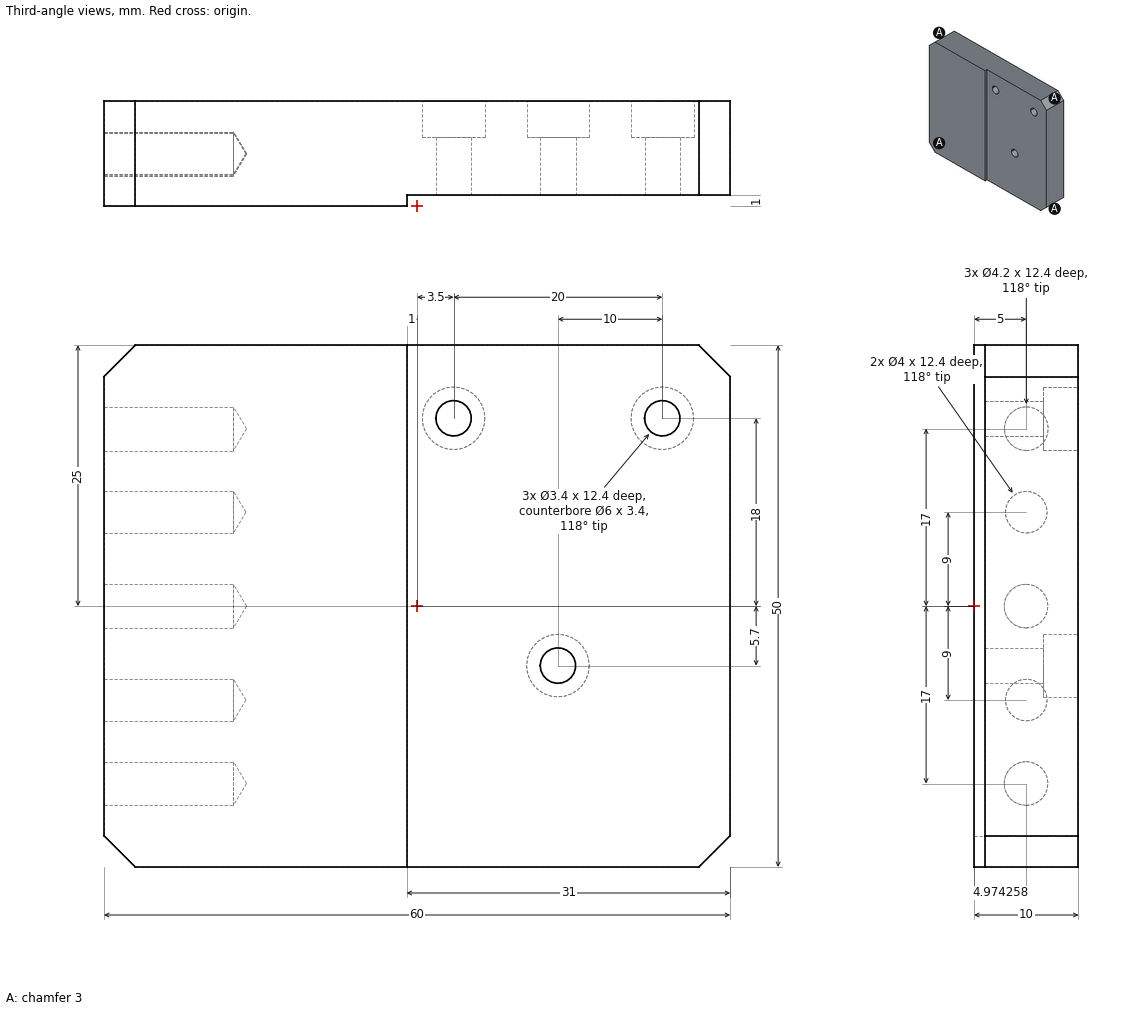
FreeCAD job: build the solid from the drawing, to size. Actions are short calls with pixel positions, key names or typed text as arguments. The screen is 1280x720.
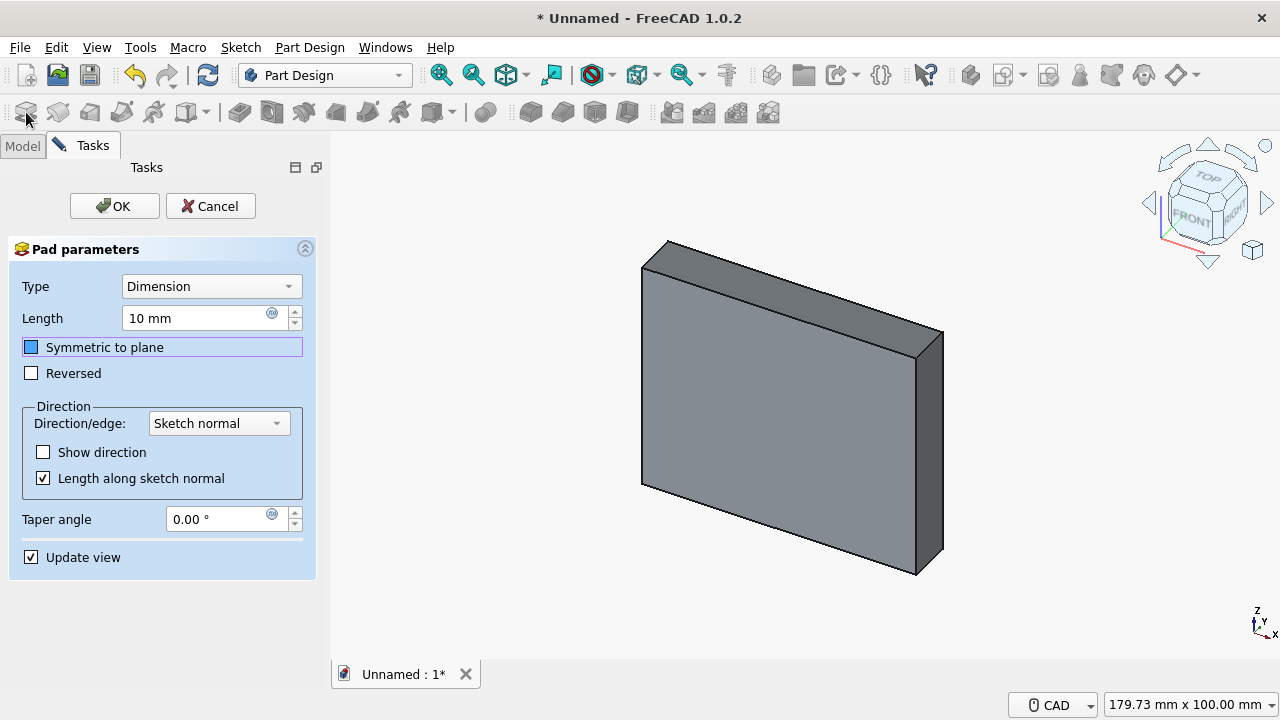
click(30, 373)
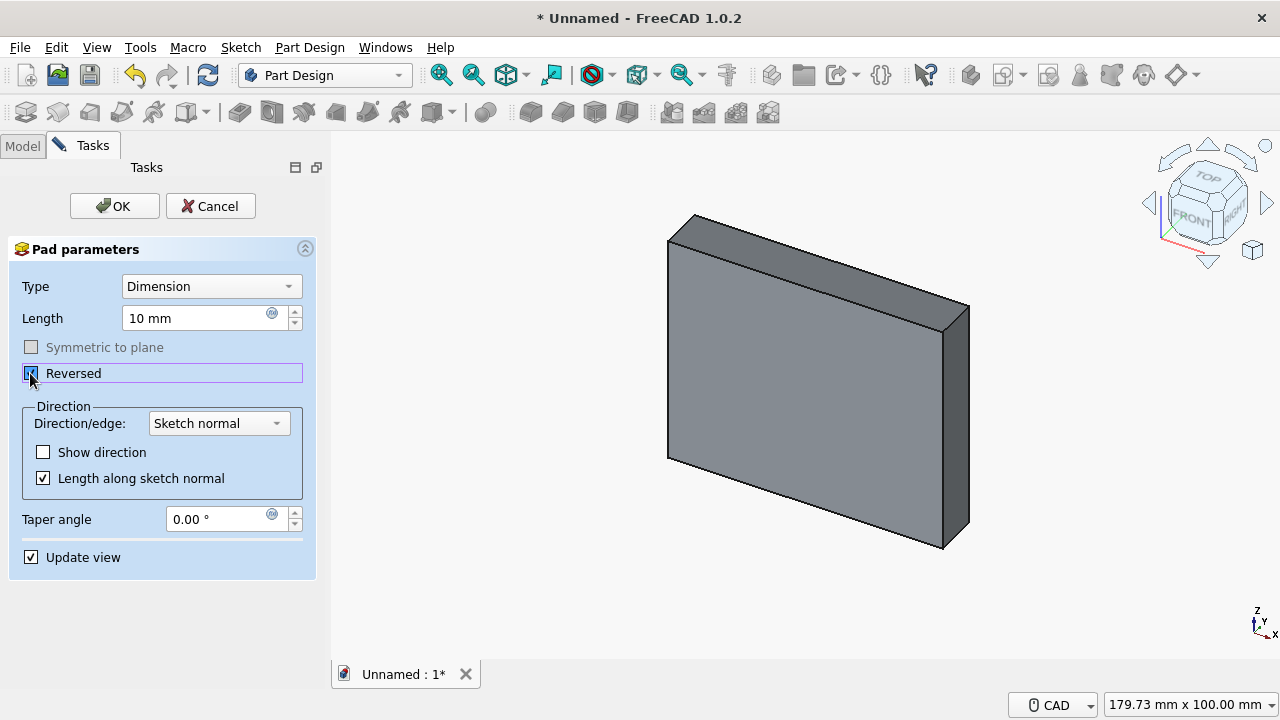
click(115, 206)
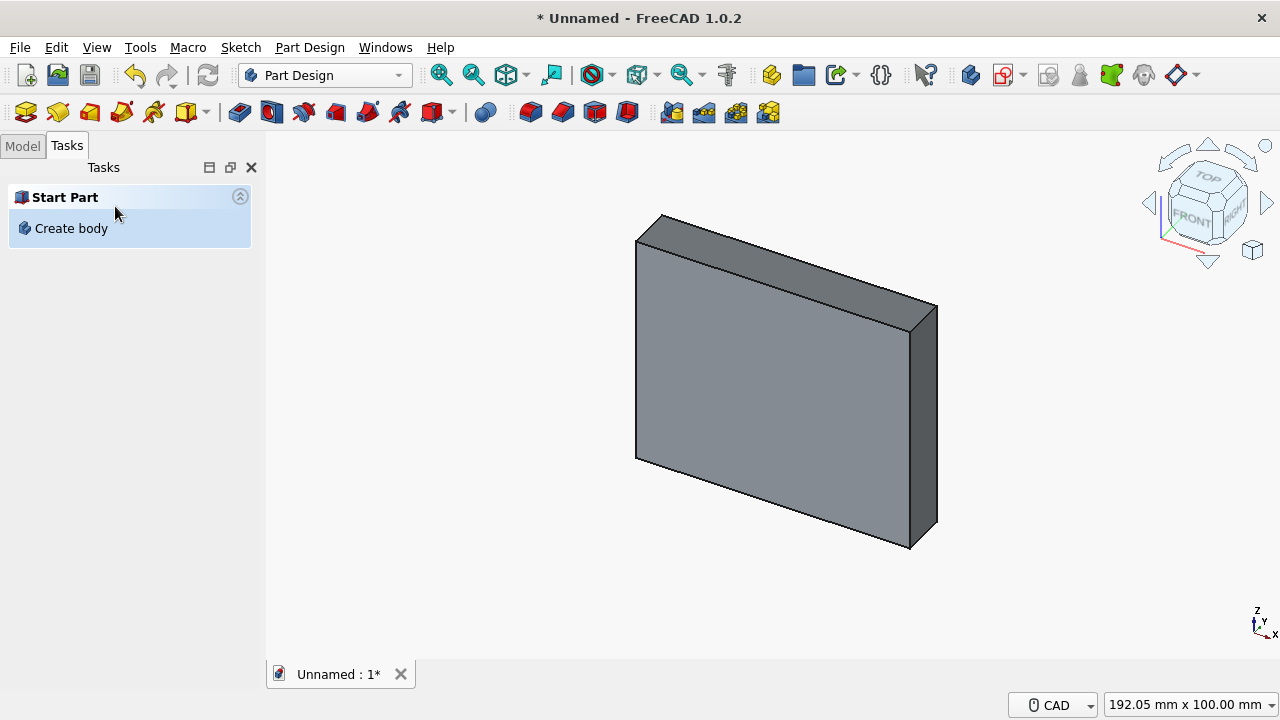
click(1004, 76)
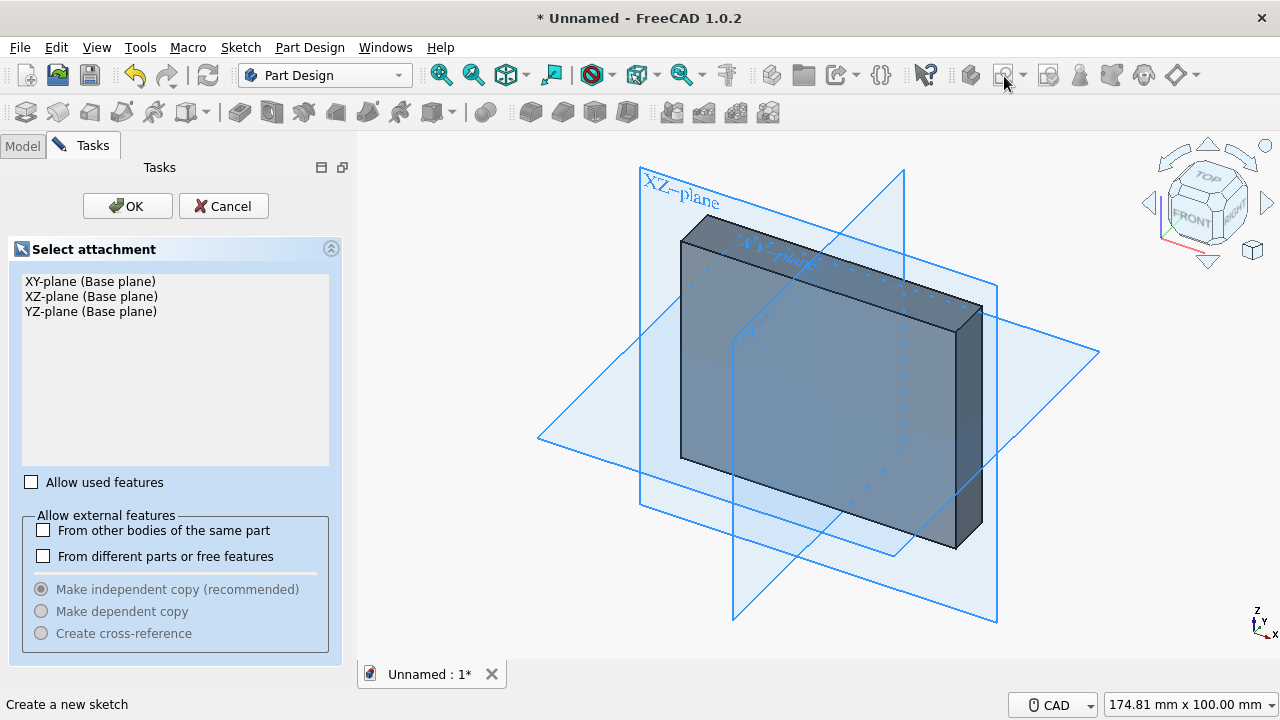
click(82, 296)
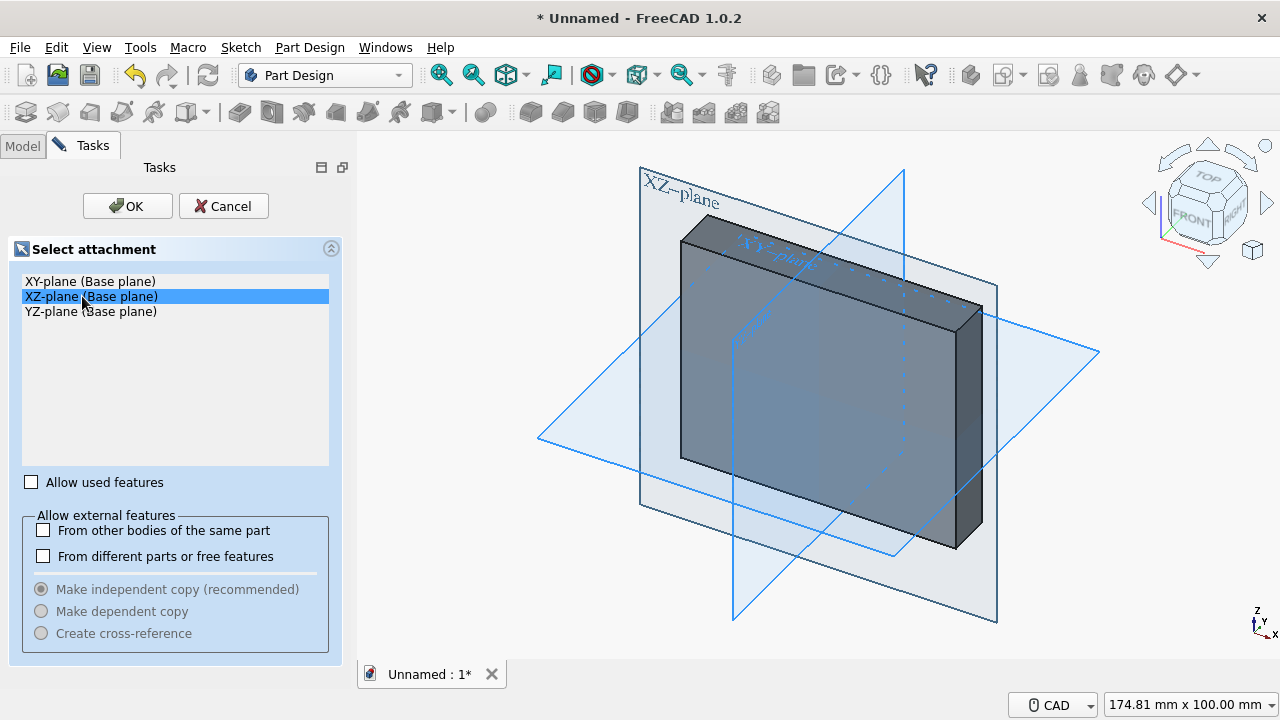
click(128, 206)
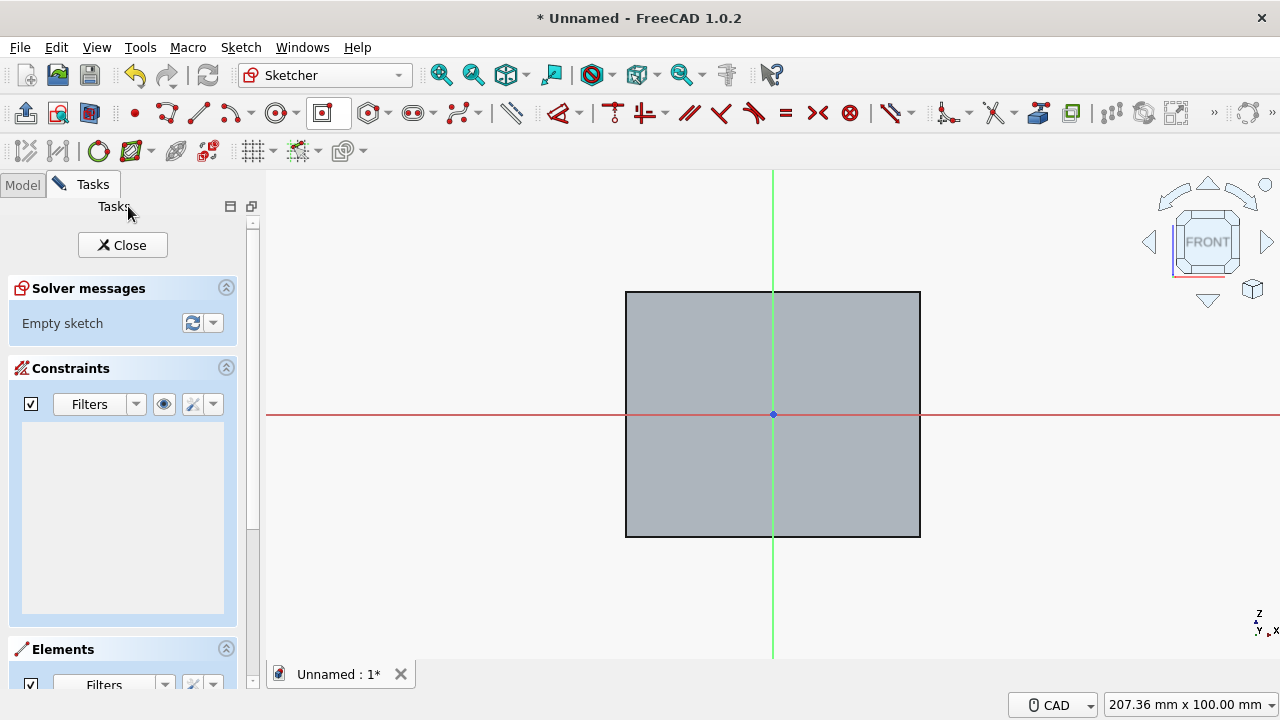
key(g)
key(r)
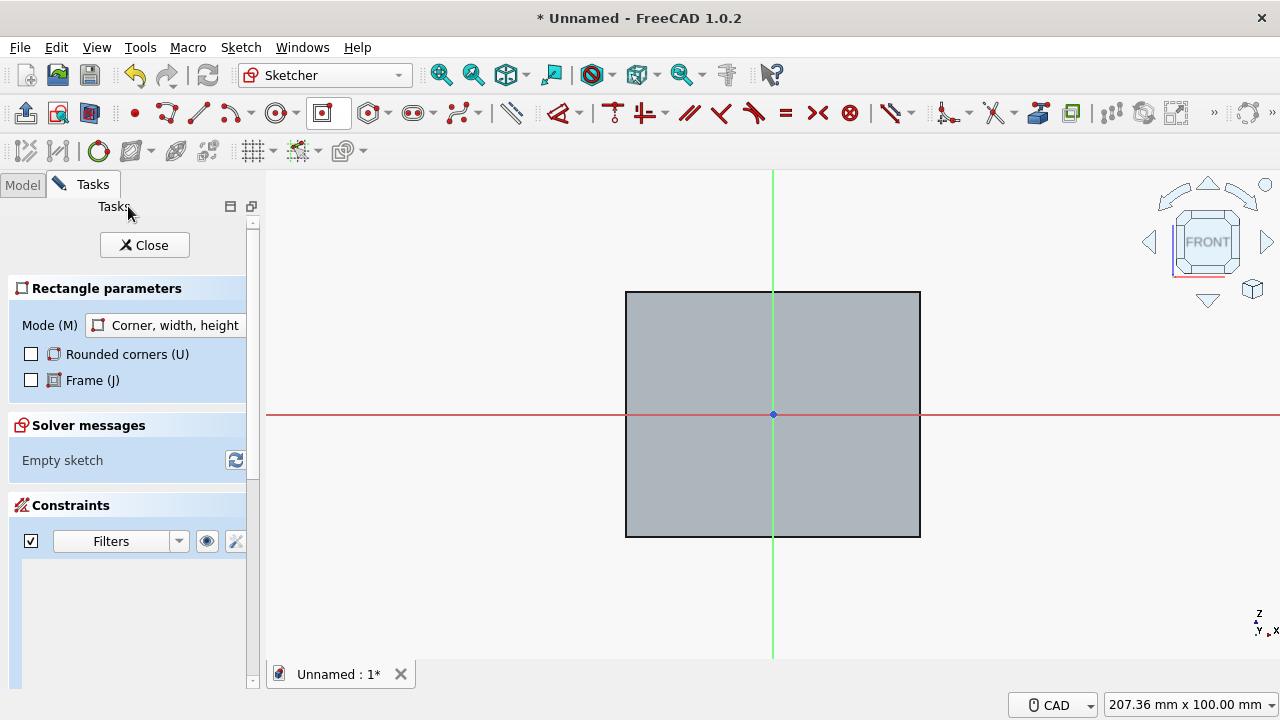
scroll(768, 292, up, 6)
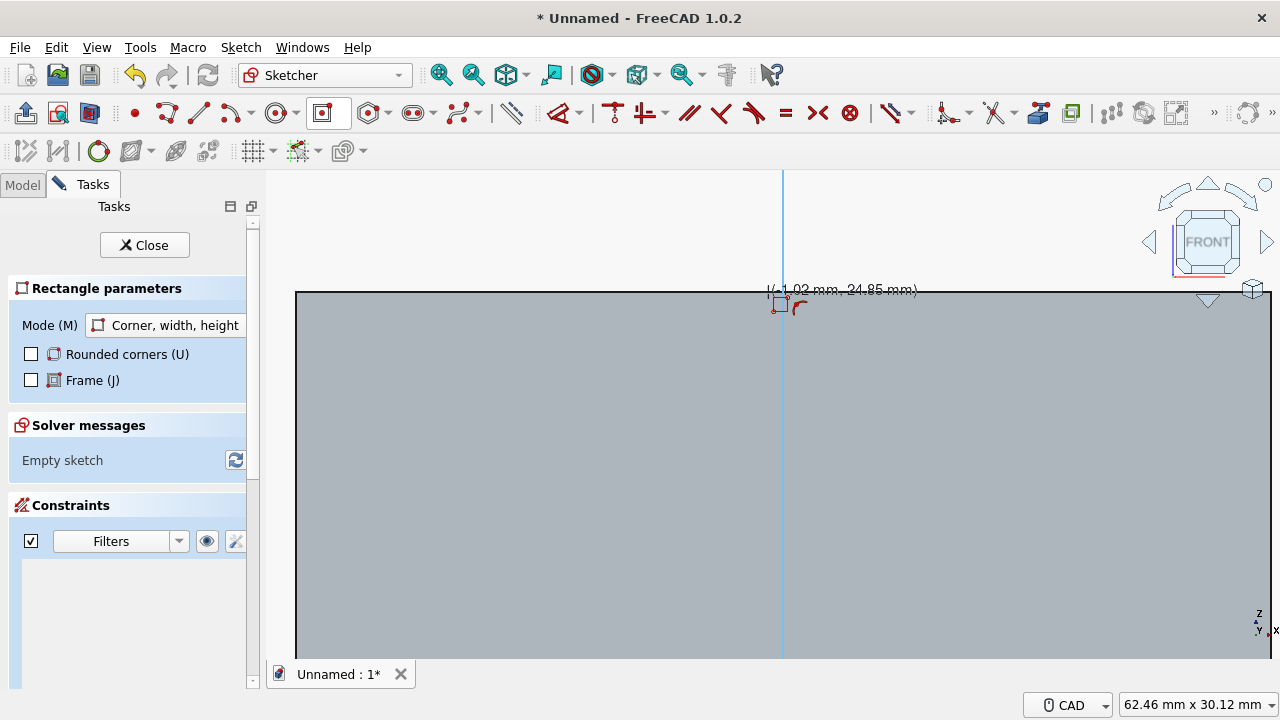
click(767, 292)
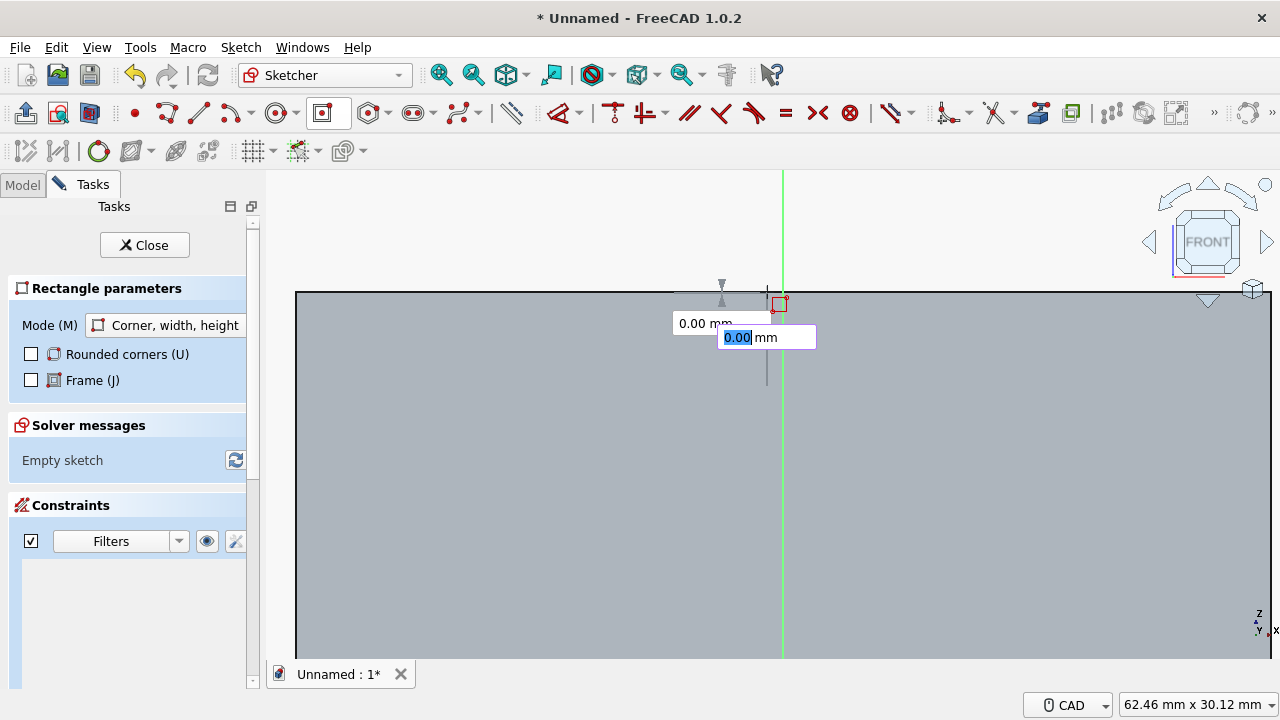
scroll(522, 249, down, 5)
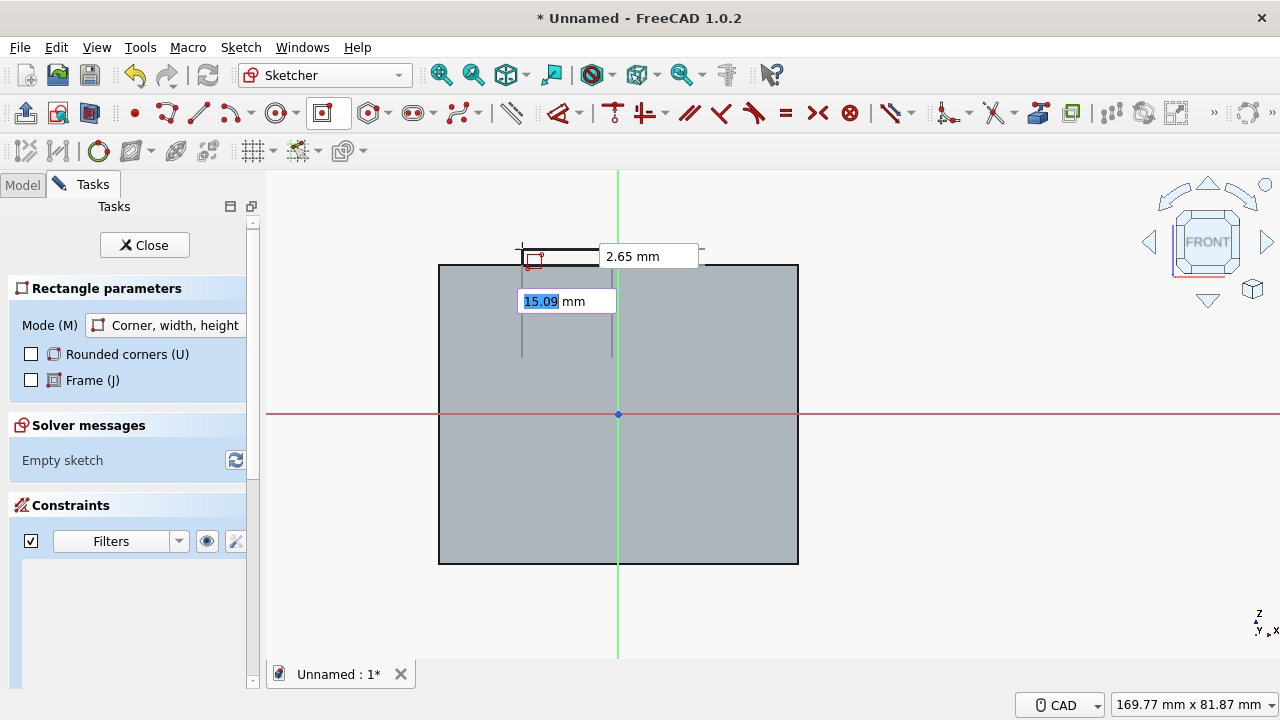
click(798, 564)
key(Escape)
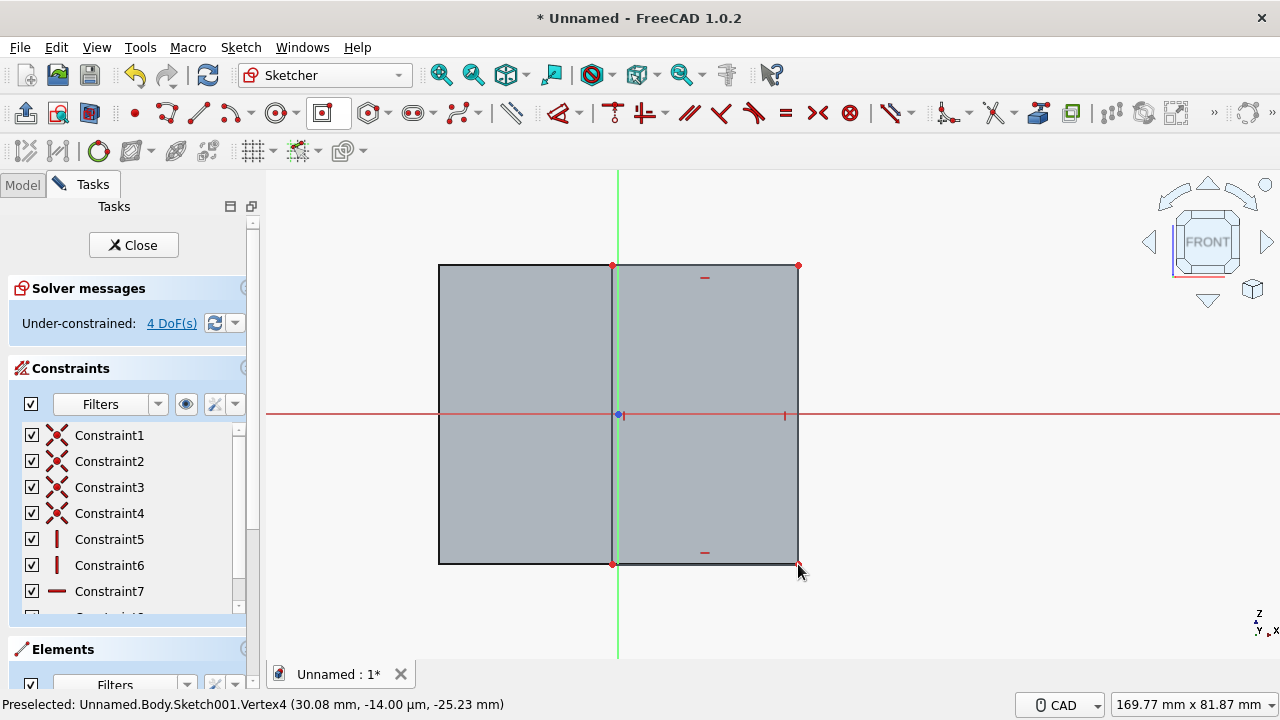
click(558, 114)